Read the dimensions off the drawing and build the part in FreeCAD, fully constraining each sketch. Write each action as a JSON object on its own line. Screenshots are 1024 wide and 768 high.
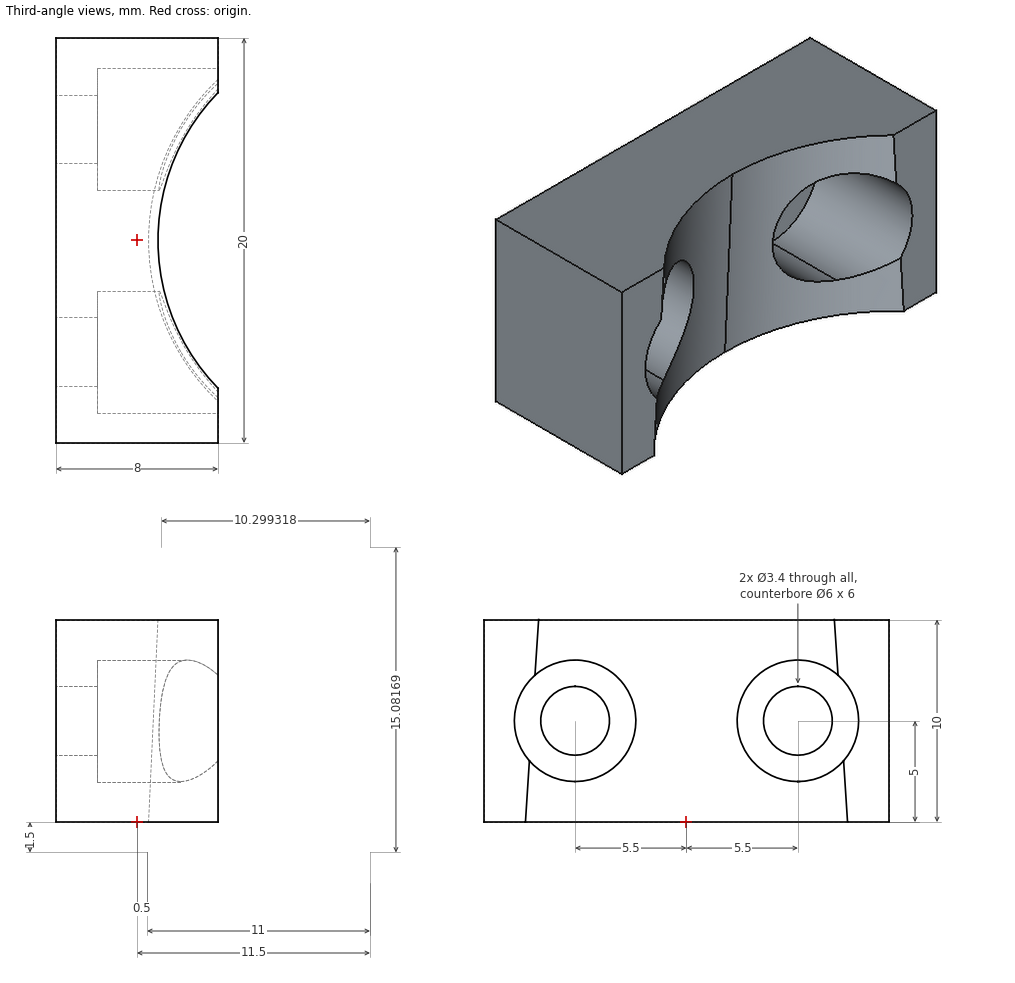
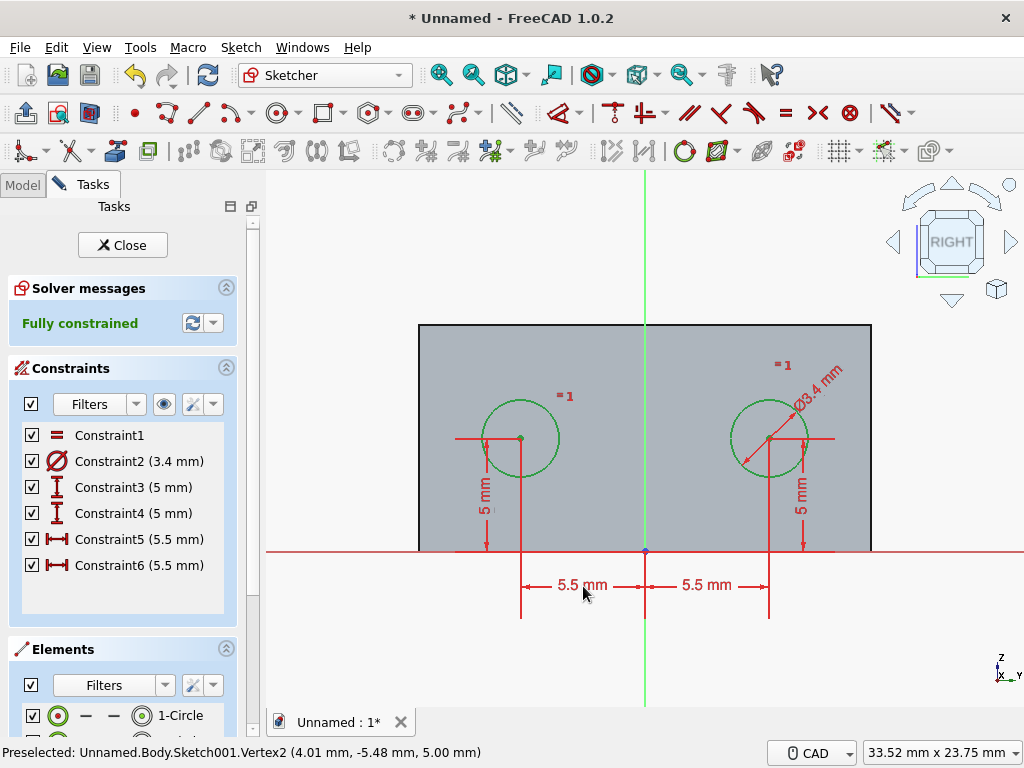
{"action": "left_click", "coordinate": [123, 245]}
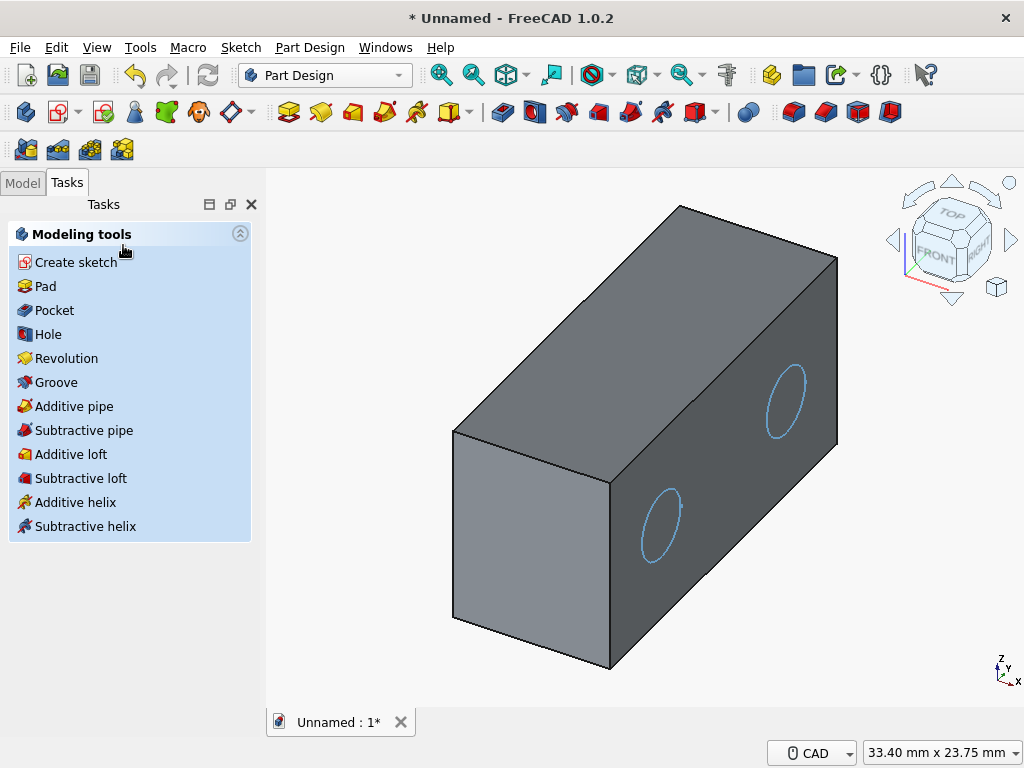
{"action": "left_click", "coordinate": [536, 112]}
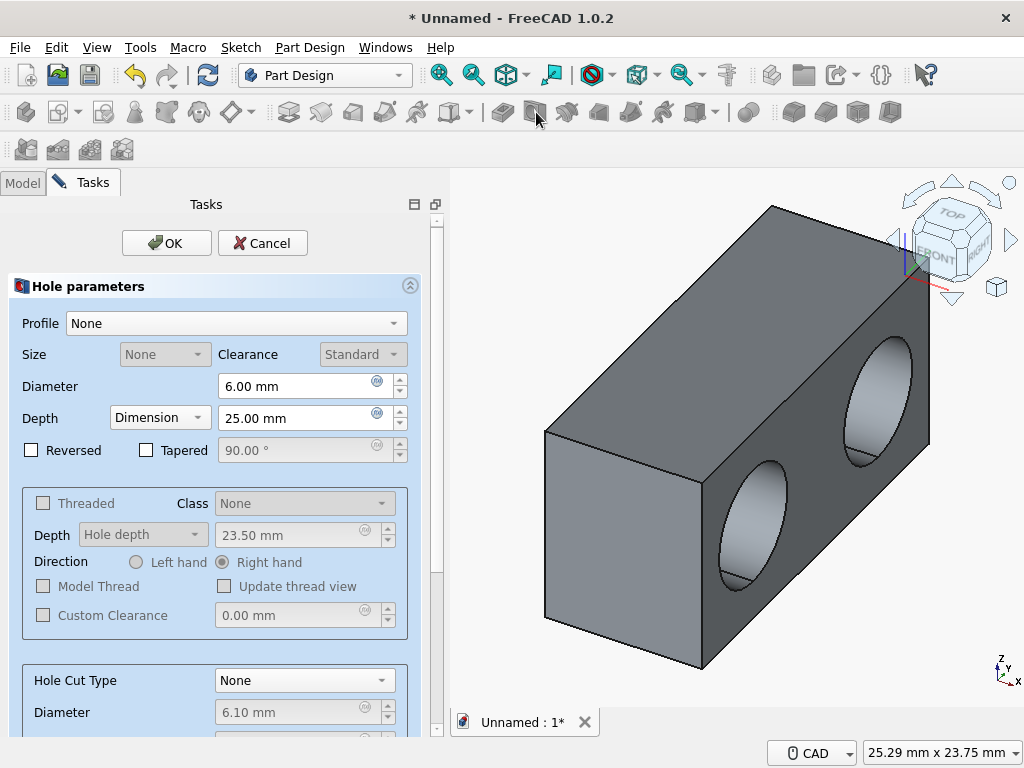
{"action": "triple_click", "coordinate": [305, 386]}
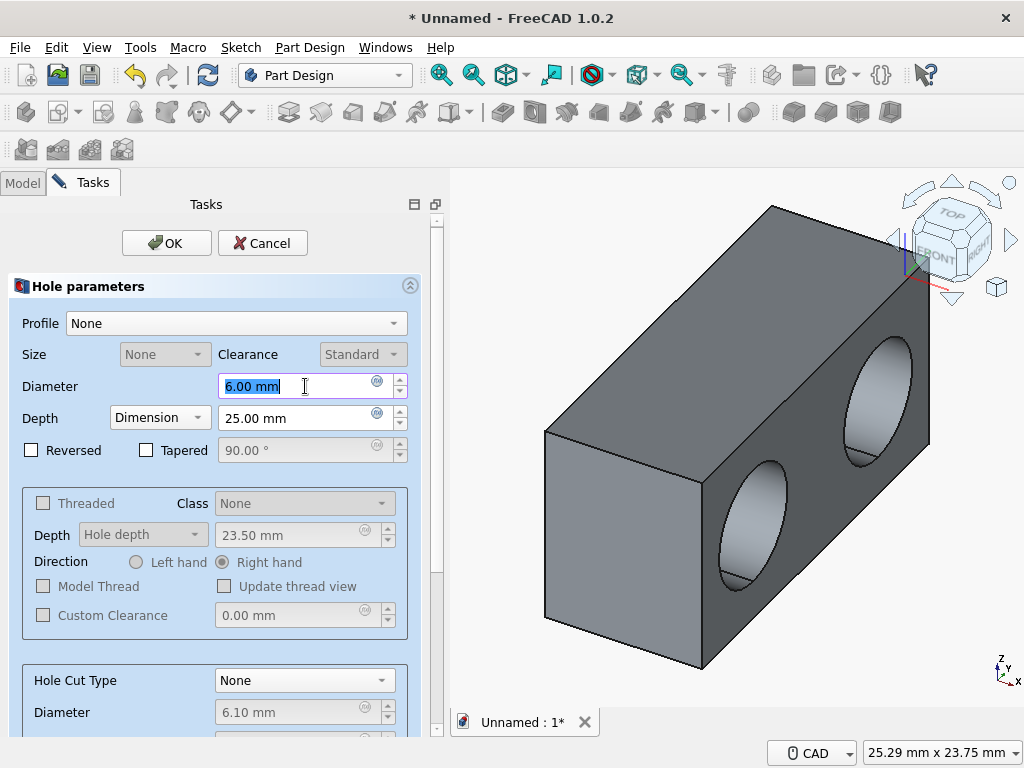
{"action": "type", "text": "3.4"}
{"action": "key", "text": "Tab"}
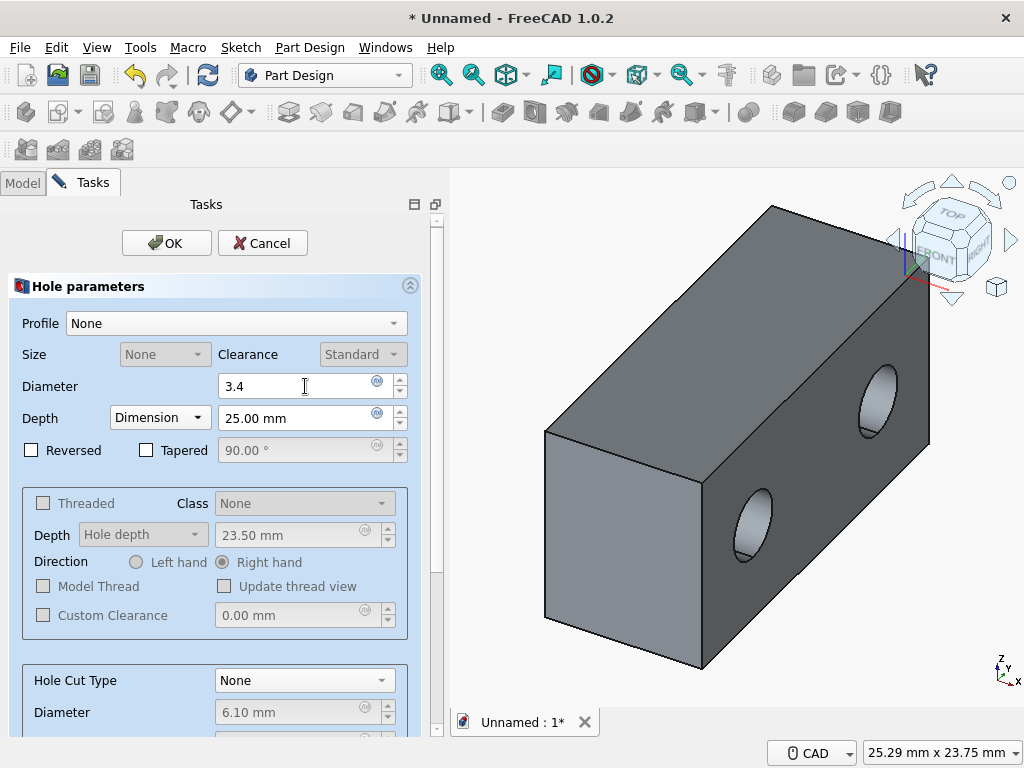
{"action": "left_click", "coordinate": [161, 418]}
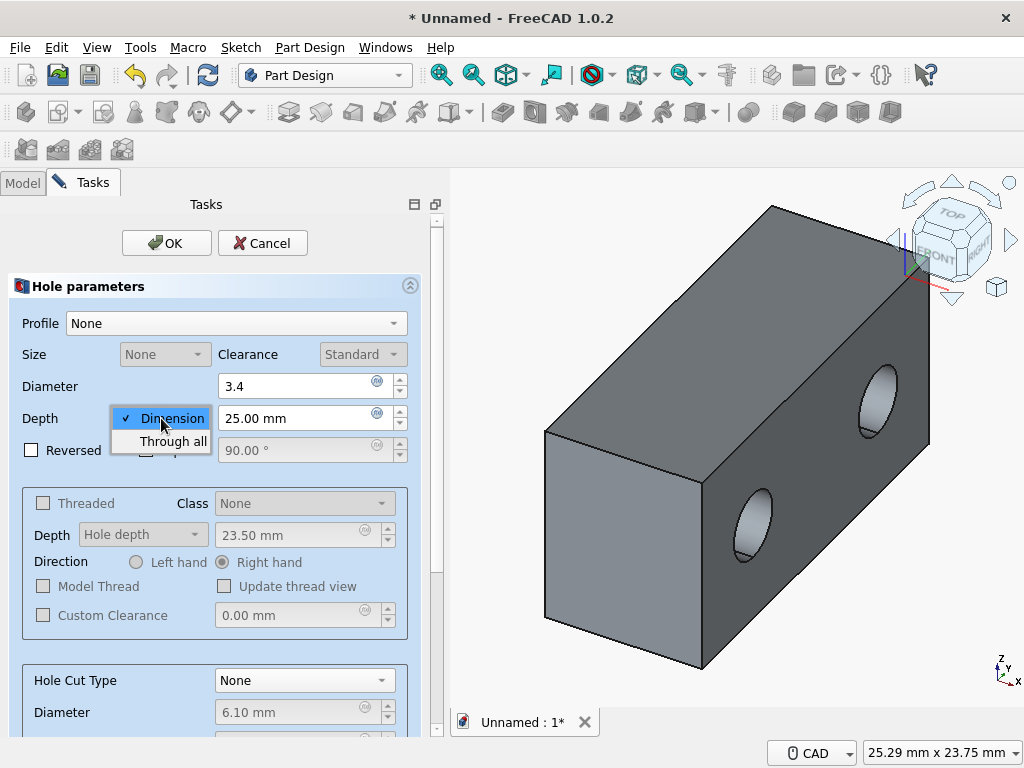
{"action": "left_click", "coordinate": [160, 442]}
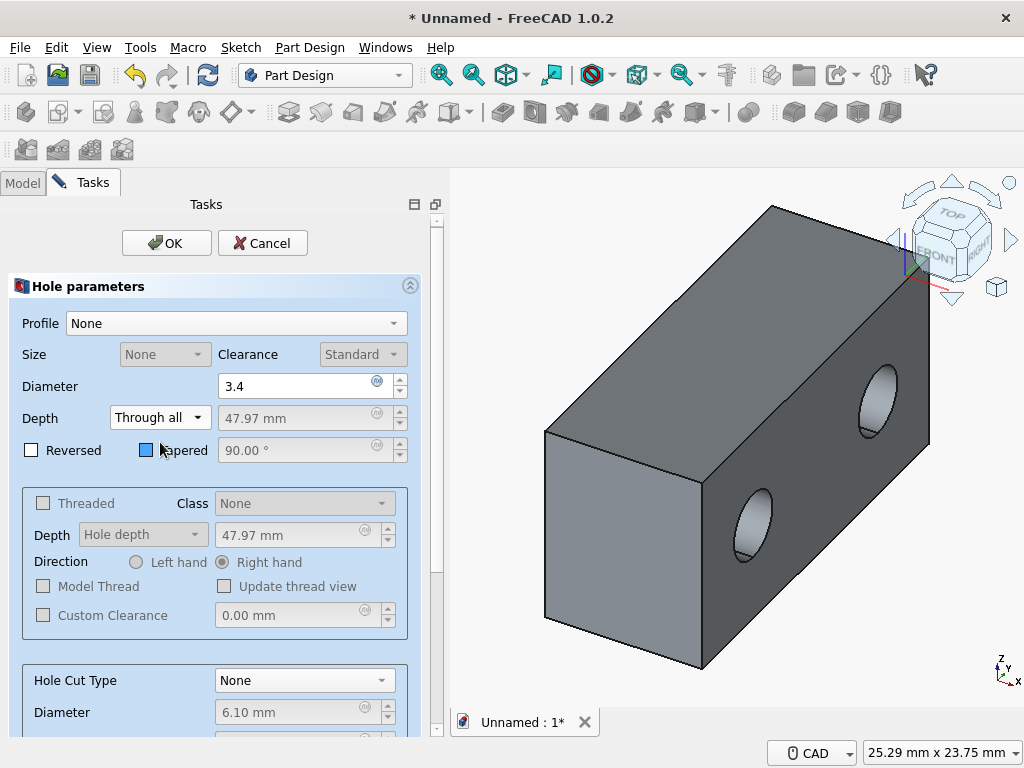
{"action": "left_click", "coordinate": [306, 680]}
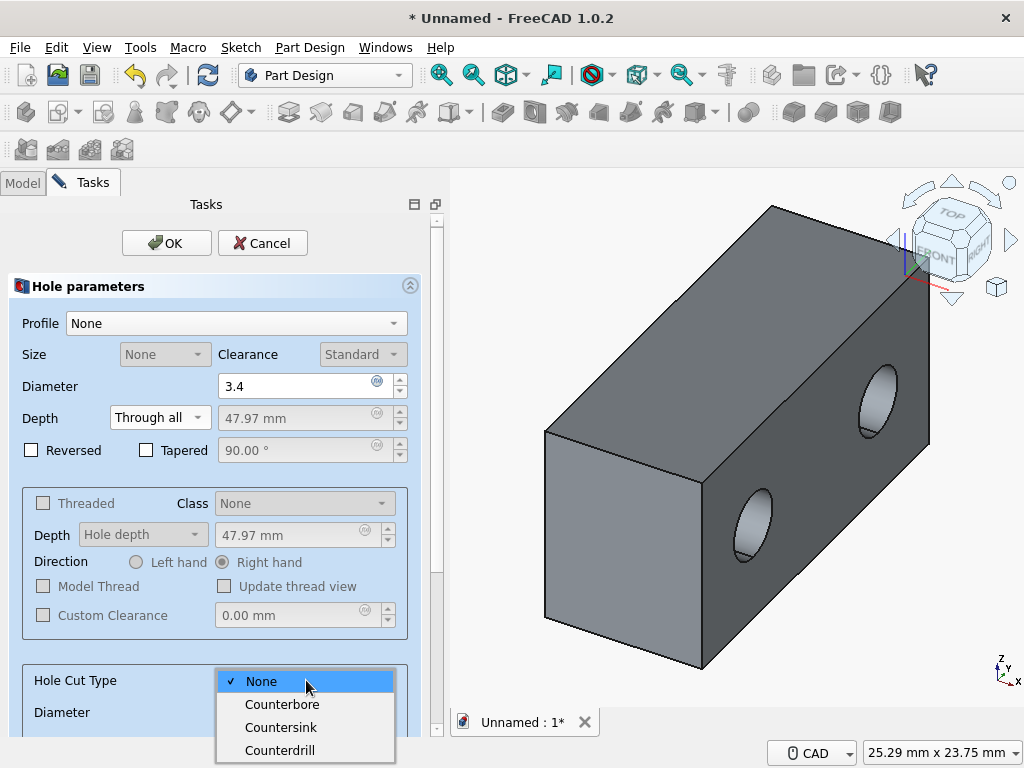
{"action": "left_click", "coordinate": [304, 704]}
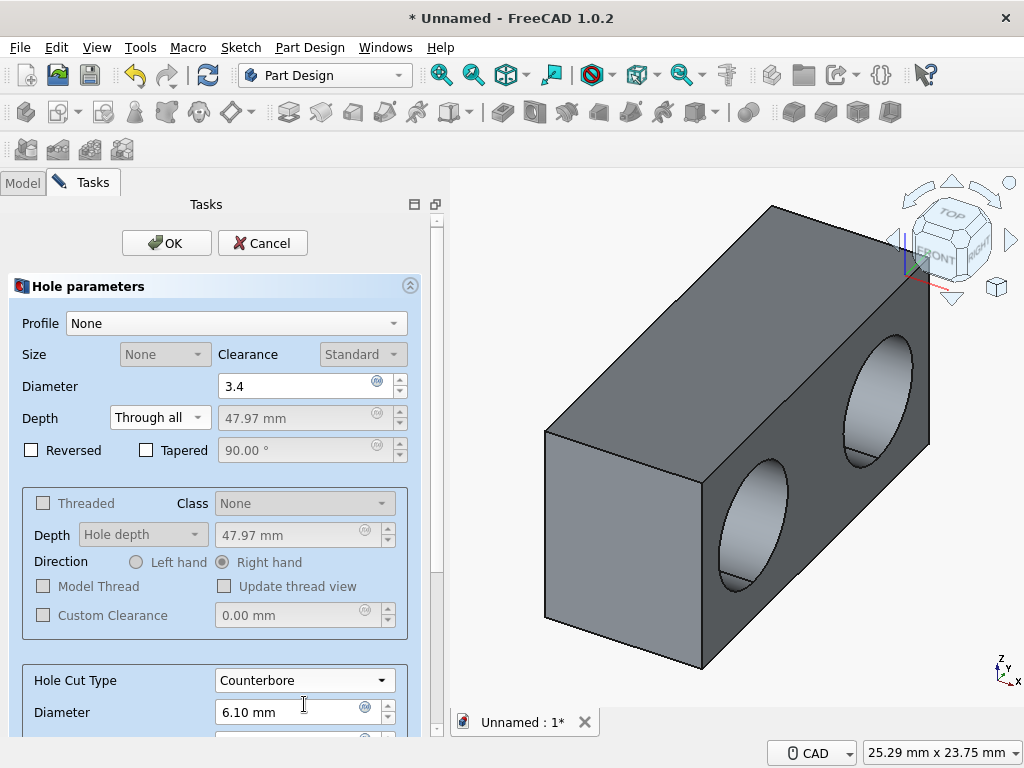
{"action": "triple_click", "coordinate": [298, 712]}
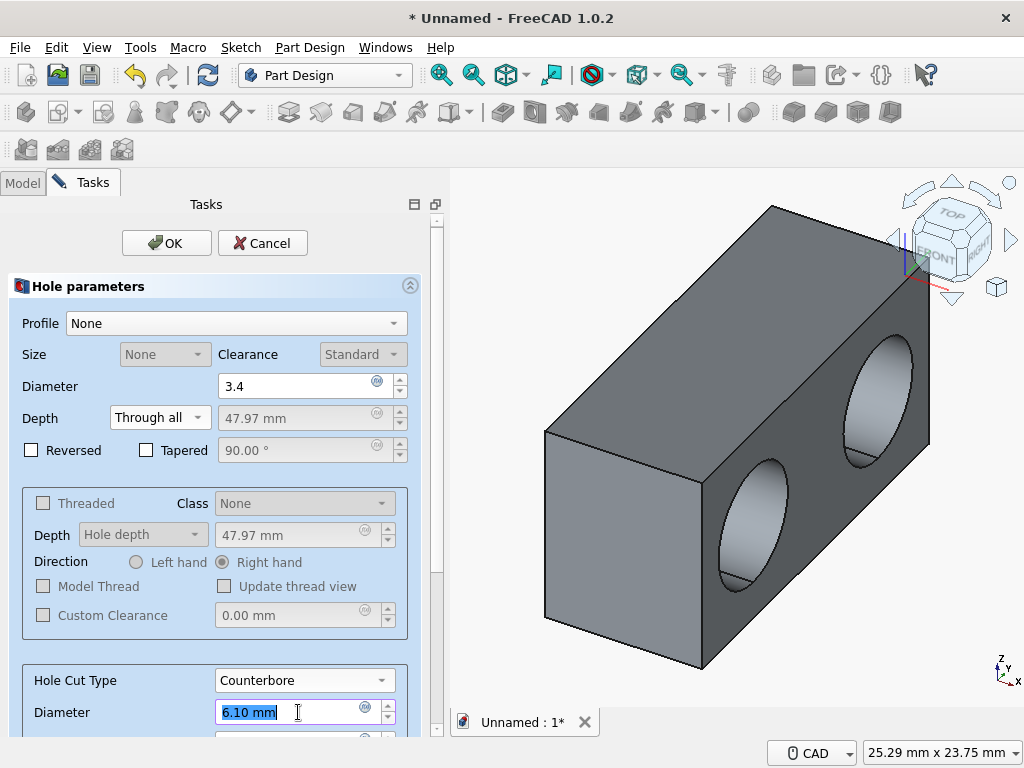
{"action": "type", "text": "6"}
{"action": "key", "text": "Tab"}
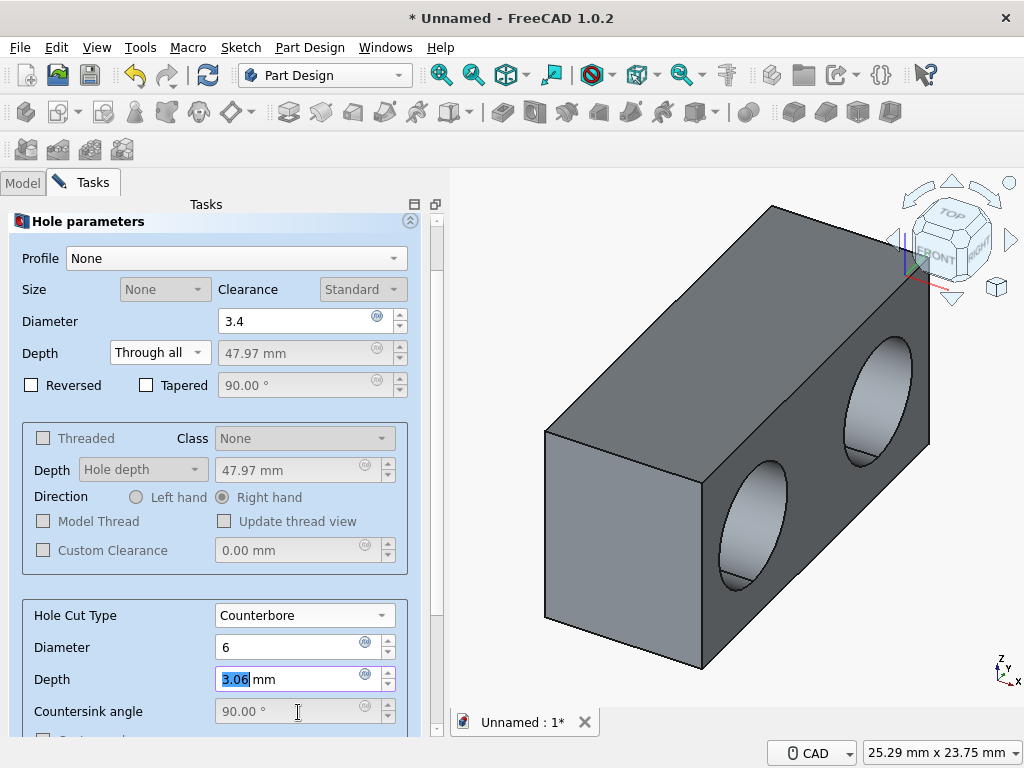
{"action": "type", "text": "6"}
{"action": "key", "text": "Tab"}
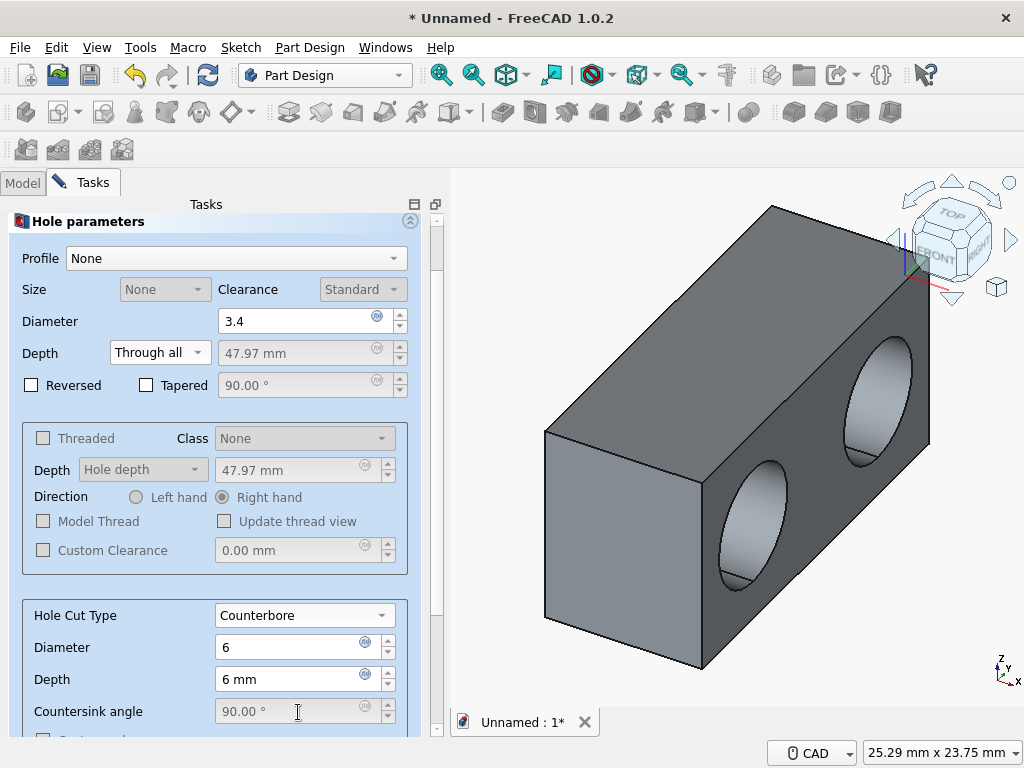
{"action": "scroll", "coordinate": [437, 475], "scroll_direction": "up", "scroll_amount": 2}